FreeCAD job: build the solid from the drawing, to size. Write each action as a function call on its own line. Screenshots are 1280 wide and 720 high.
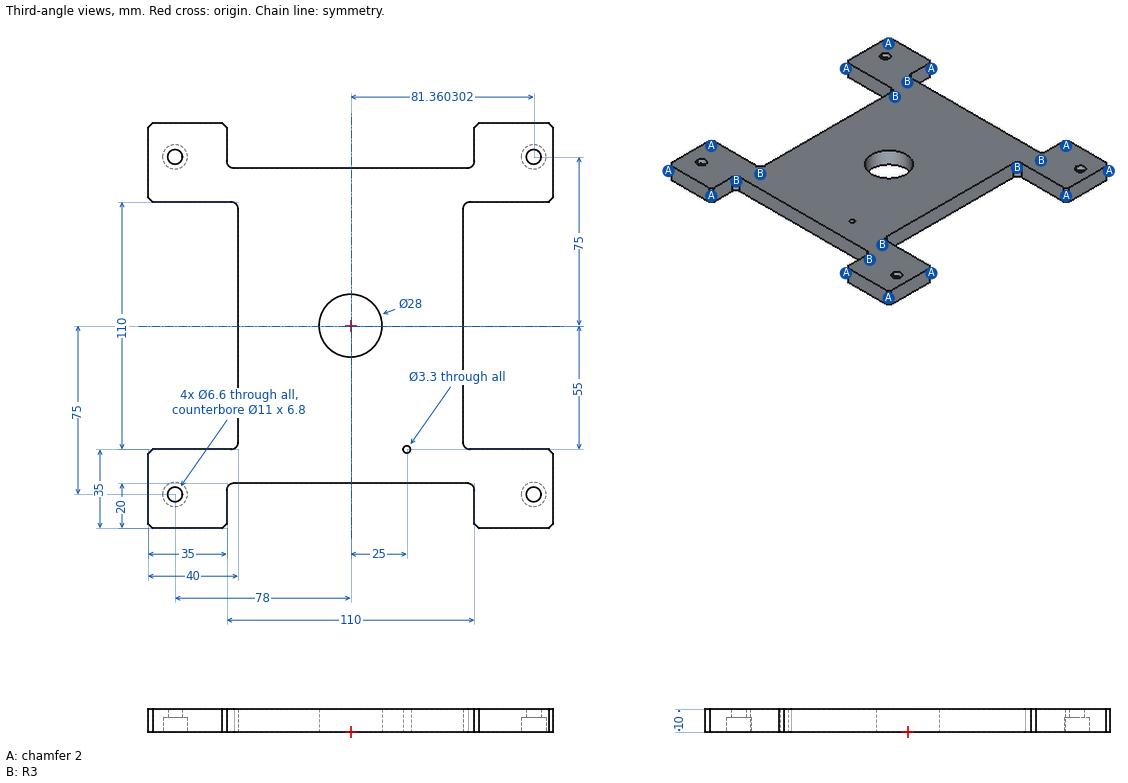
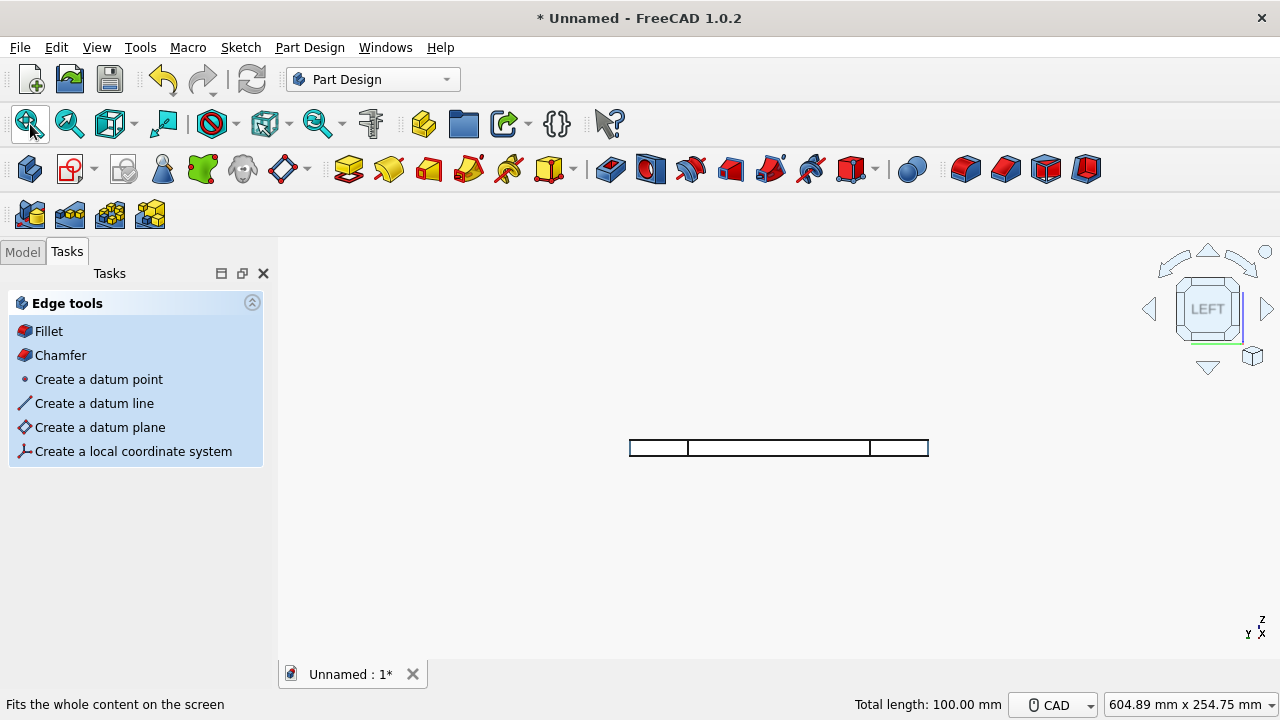
click(688, 447, ctrl)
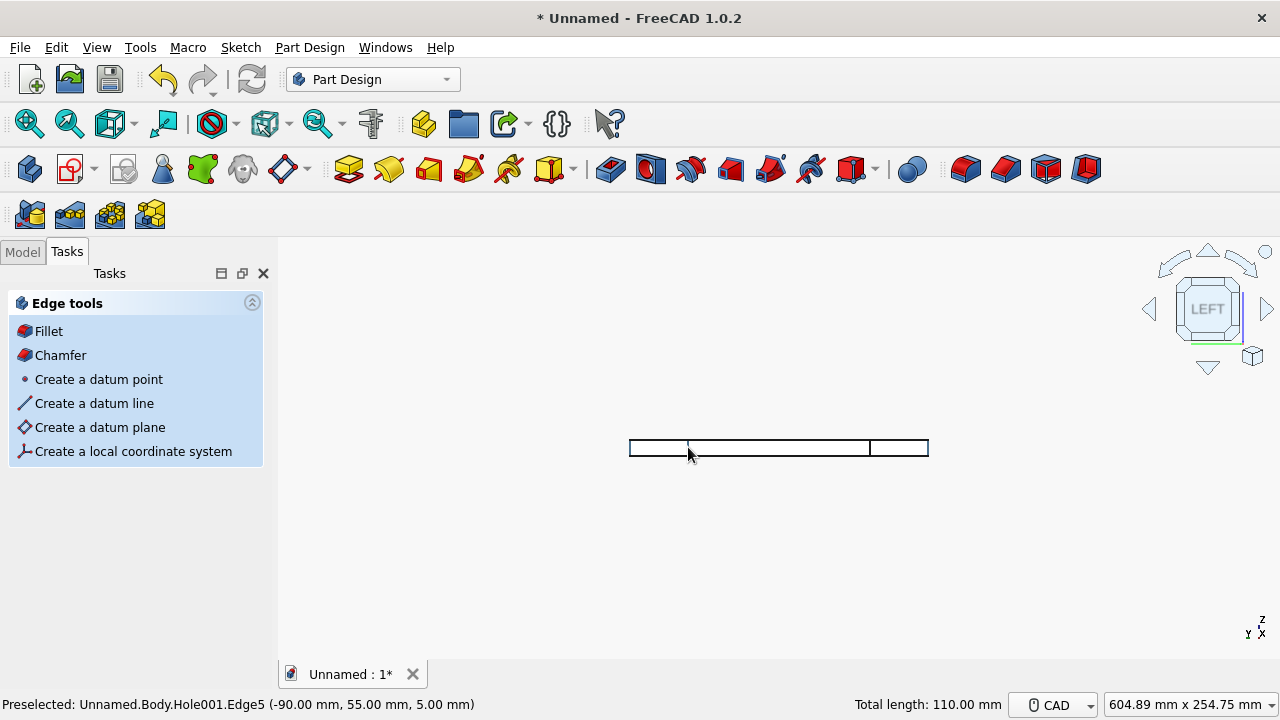
click(870, 447, ctrl)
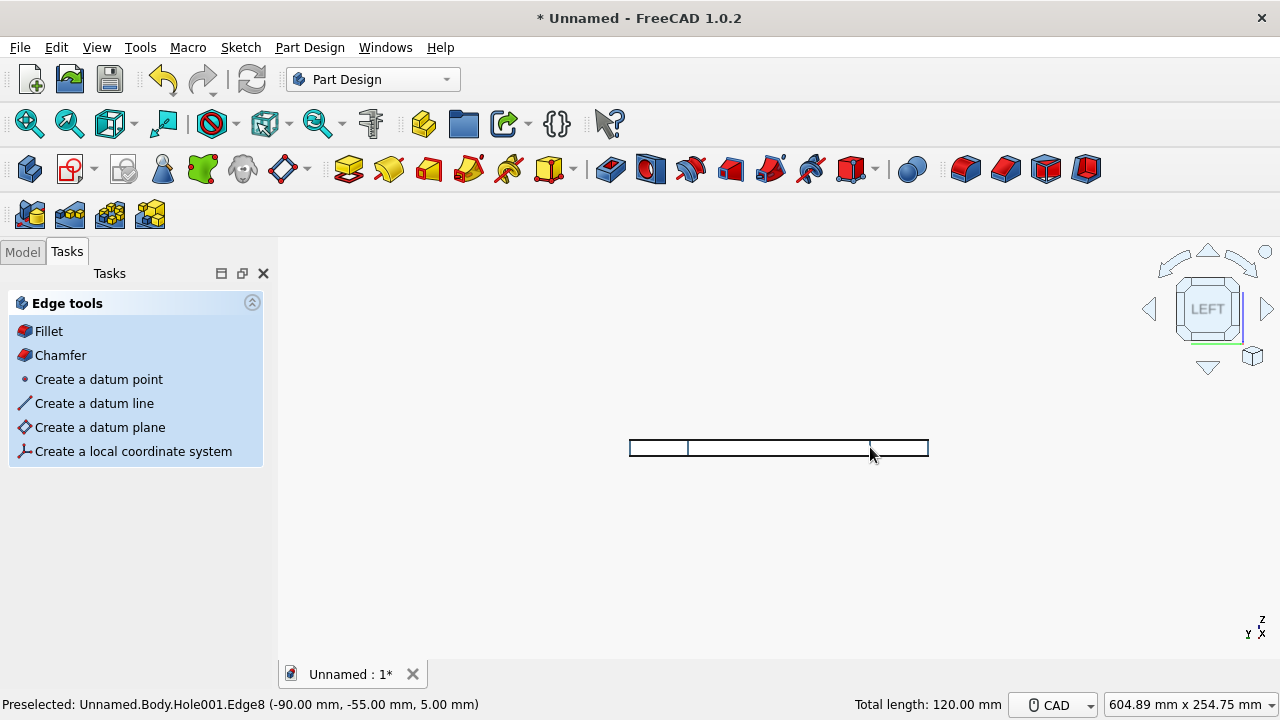
click(1006, 170)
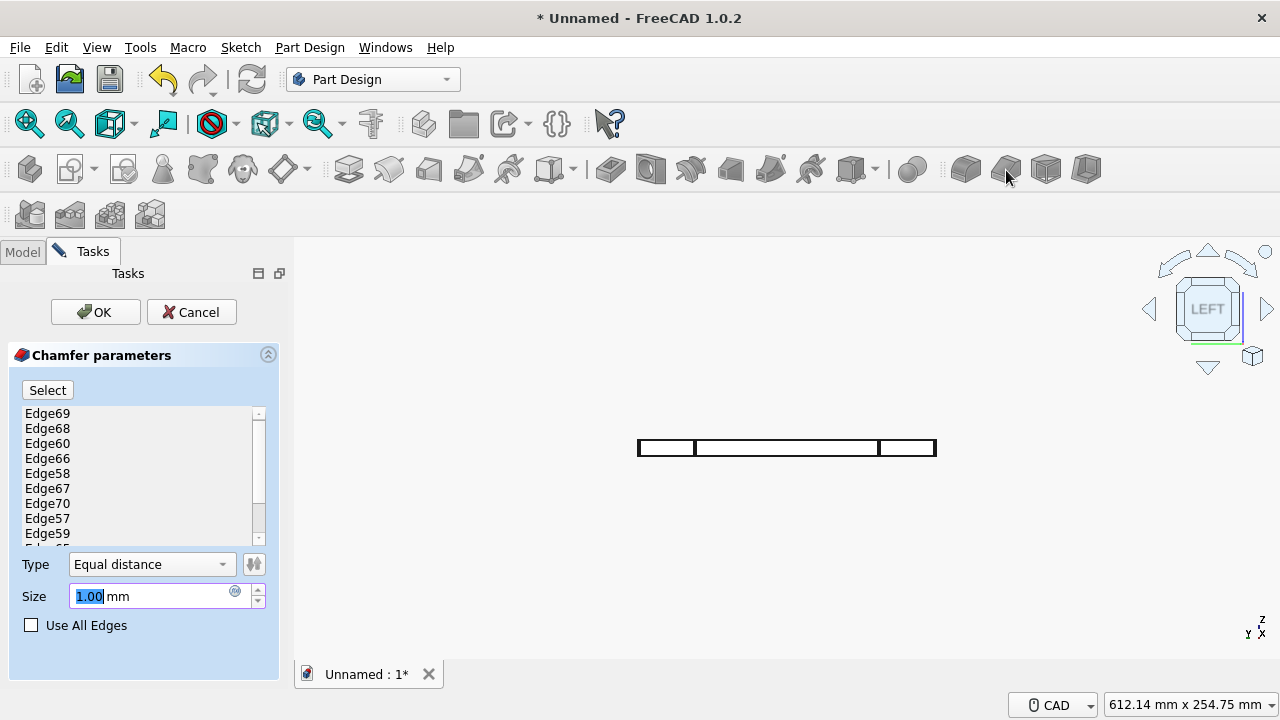
text(2)
key(Tab)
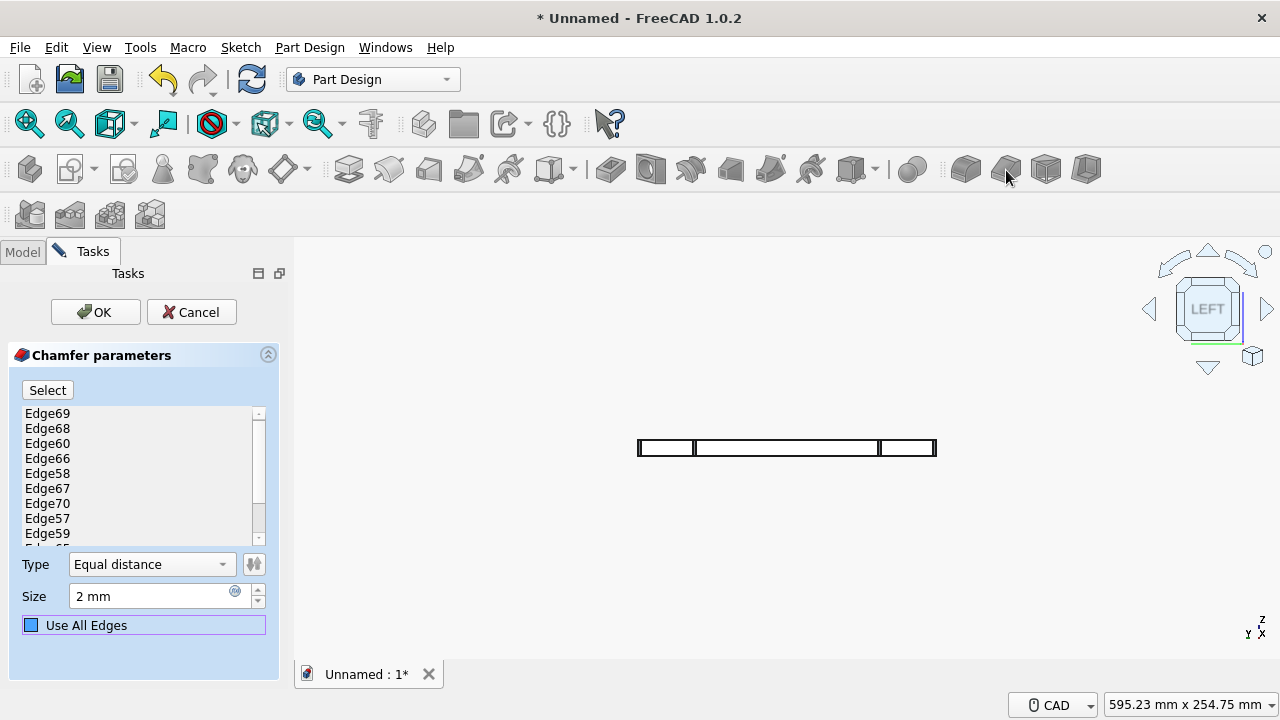
click(96, 312)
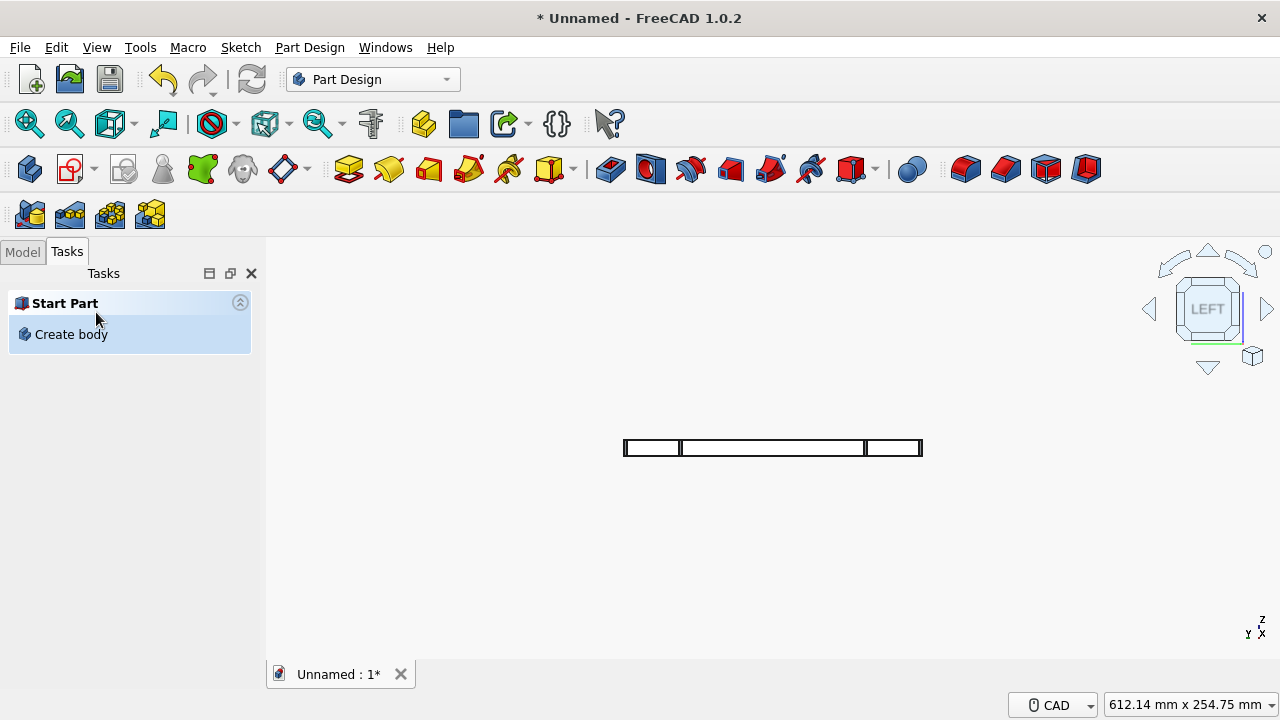
click(30, 124)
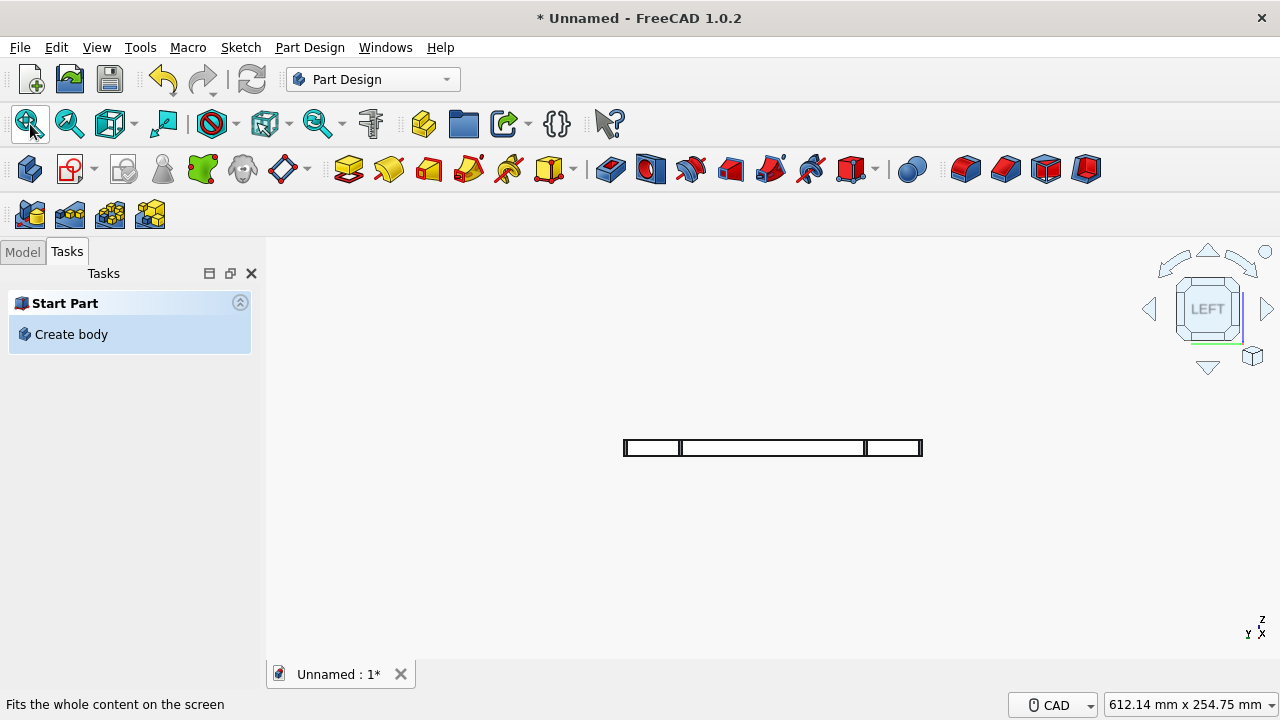
scroll(657, 447, up, 5)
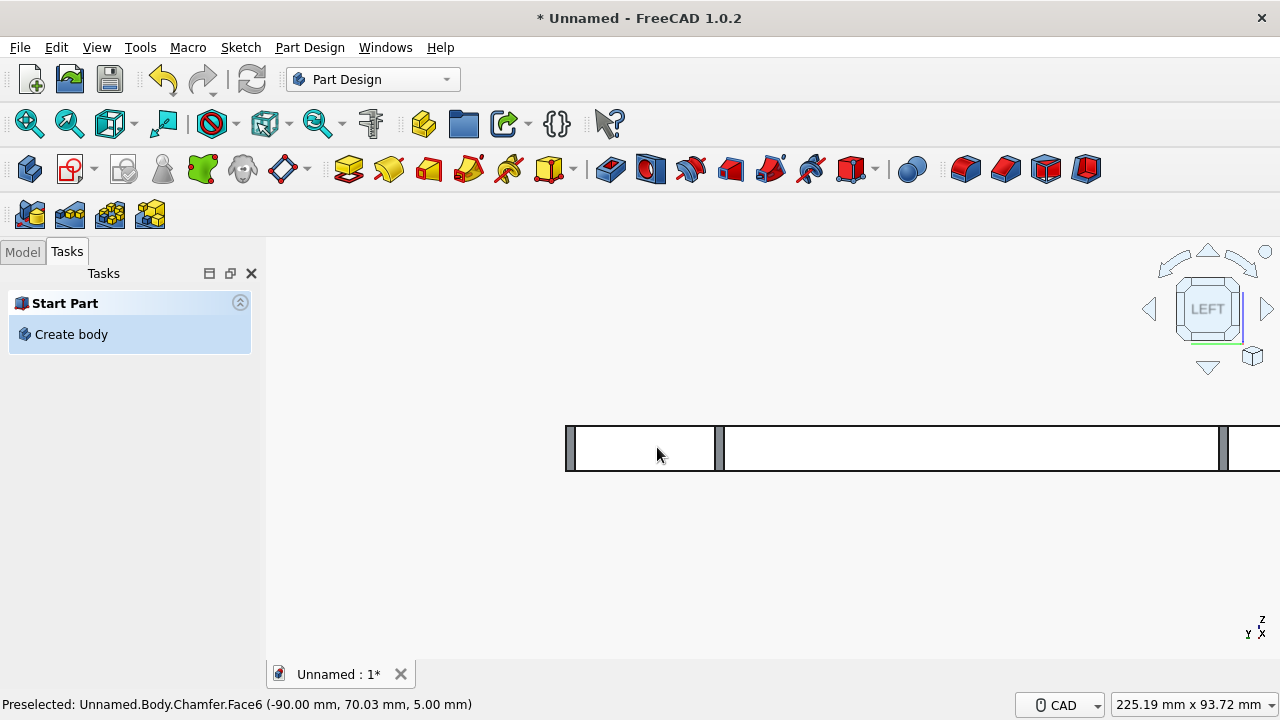
click(30, 124)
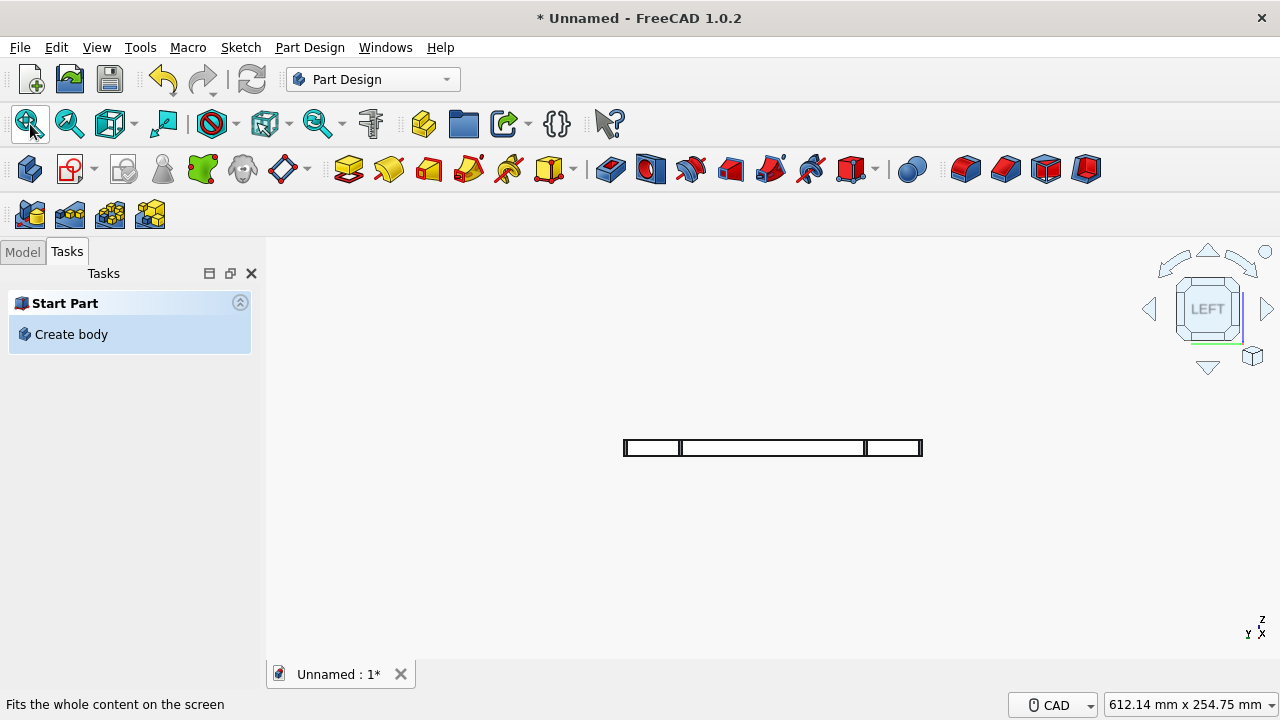
key(0)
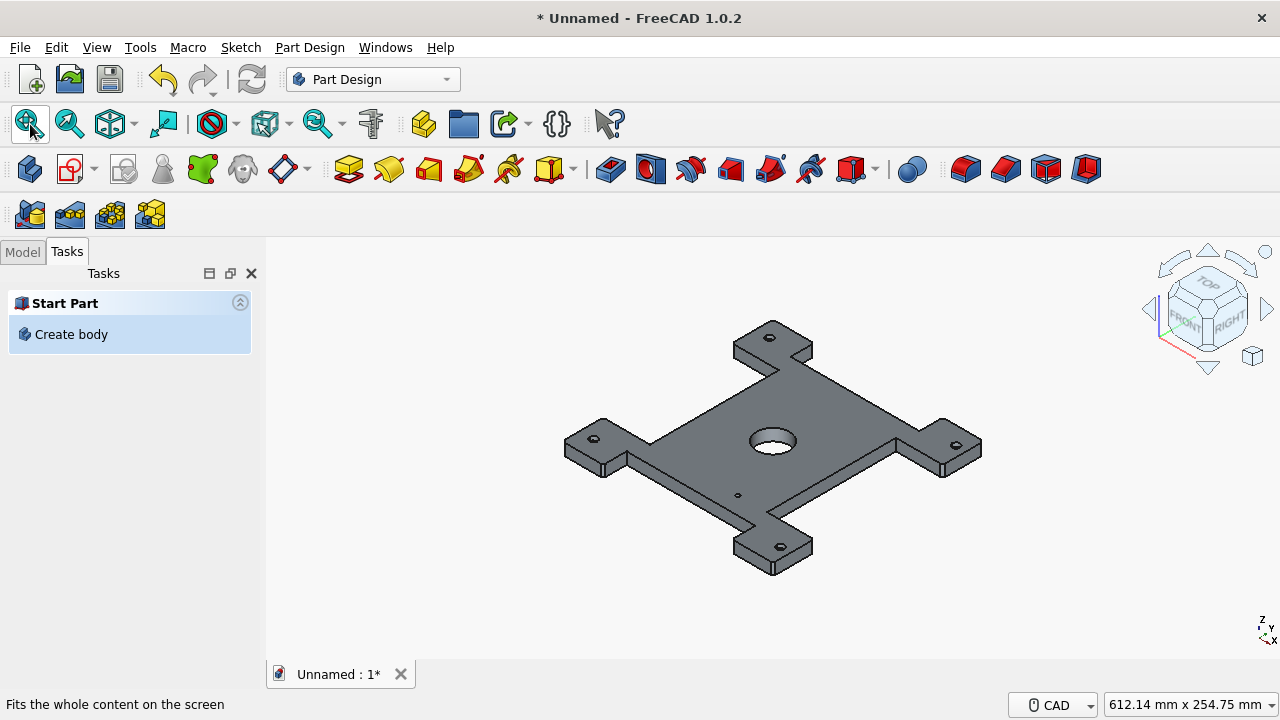
scroll(791, 362, up, 5)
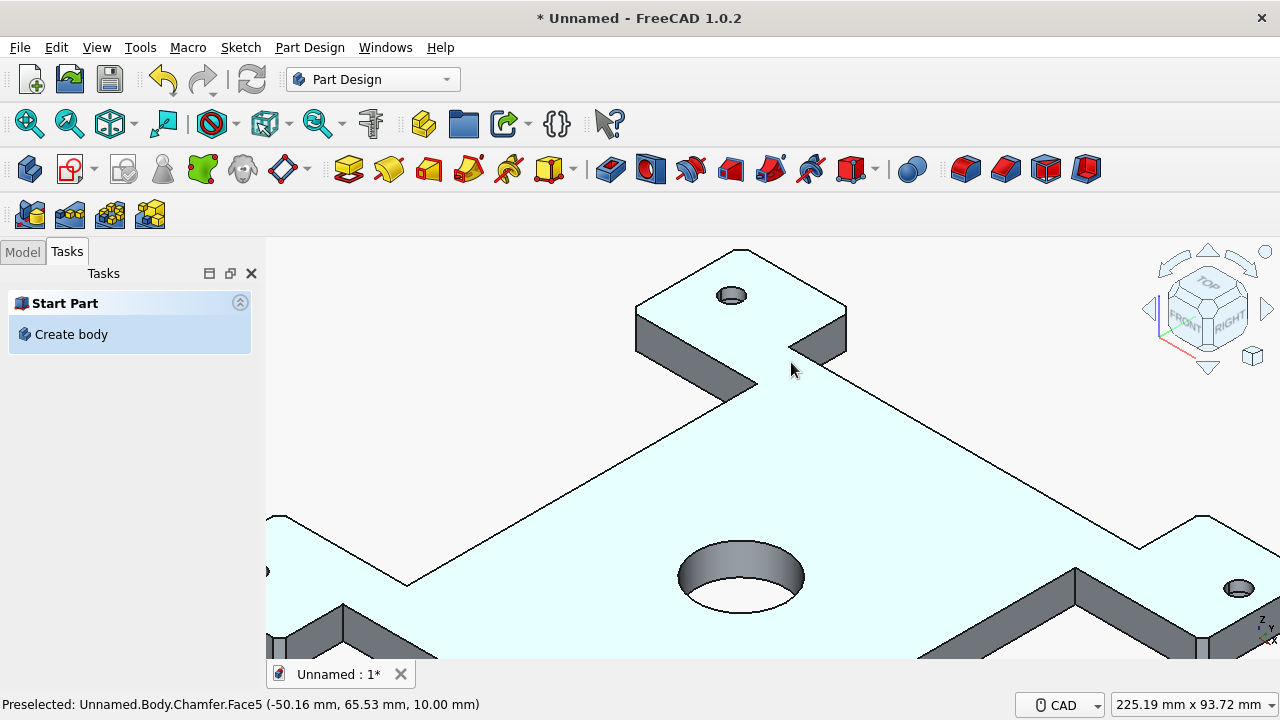
click(30, 124)